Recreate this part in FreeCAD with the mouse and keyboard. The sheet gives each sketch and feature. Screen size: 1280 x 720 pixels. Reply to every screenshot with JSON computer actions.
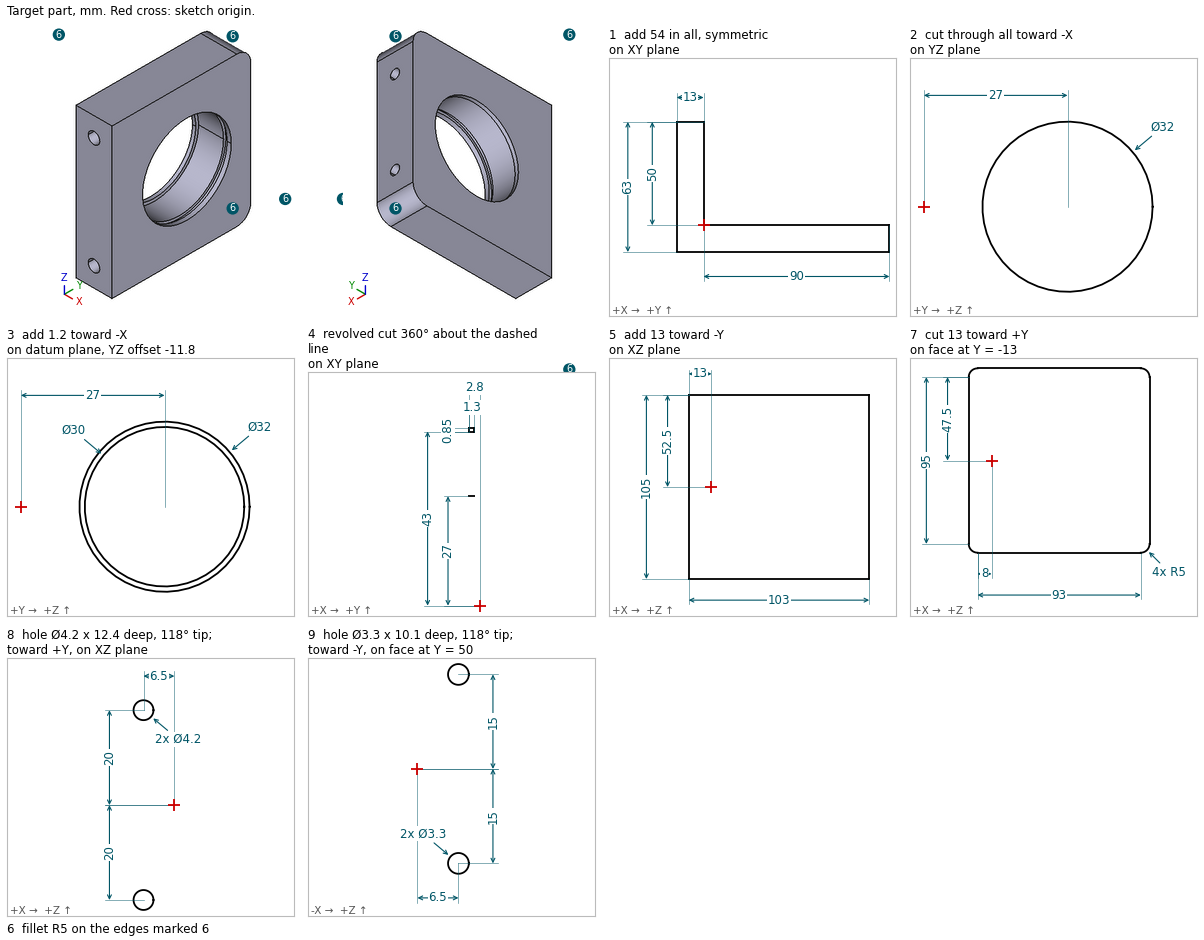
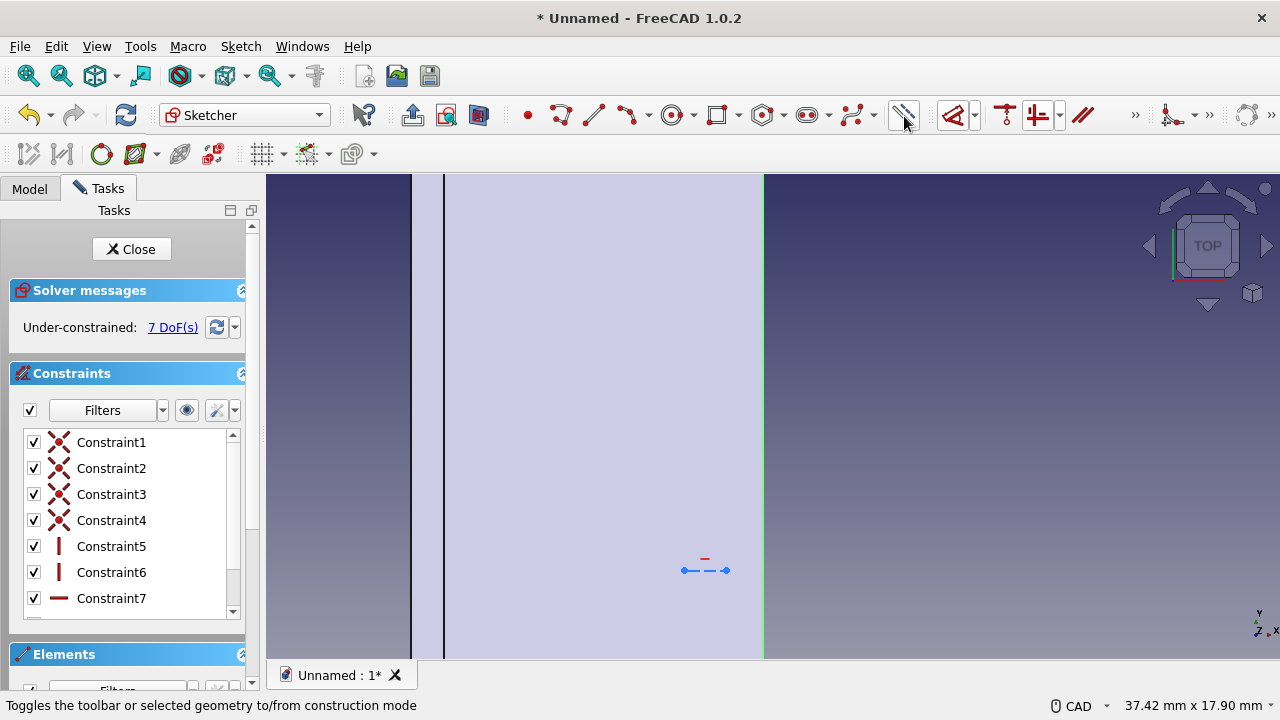
{"action": "scroll", "coordinate": [703, 571], "scroll_direction": "down", "scroll_amount": 2}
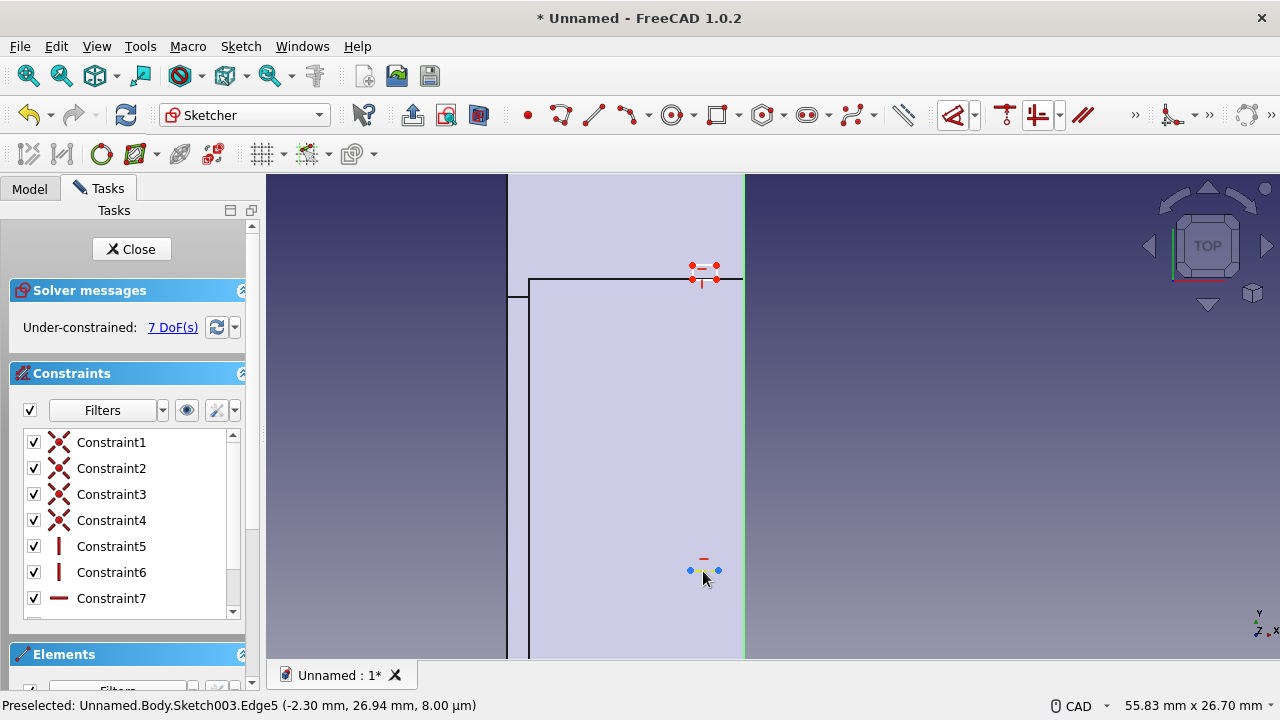
{"action": "scroll", "coordinate": [700, 280], "scroll_direction": "up", "scroll_amount": 4}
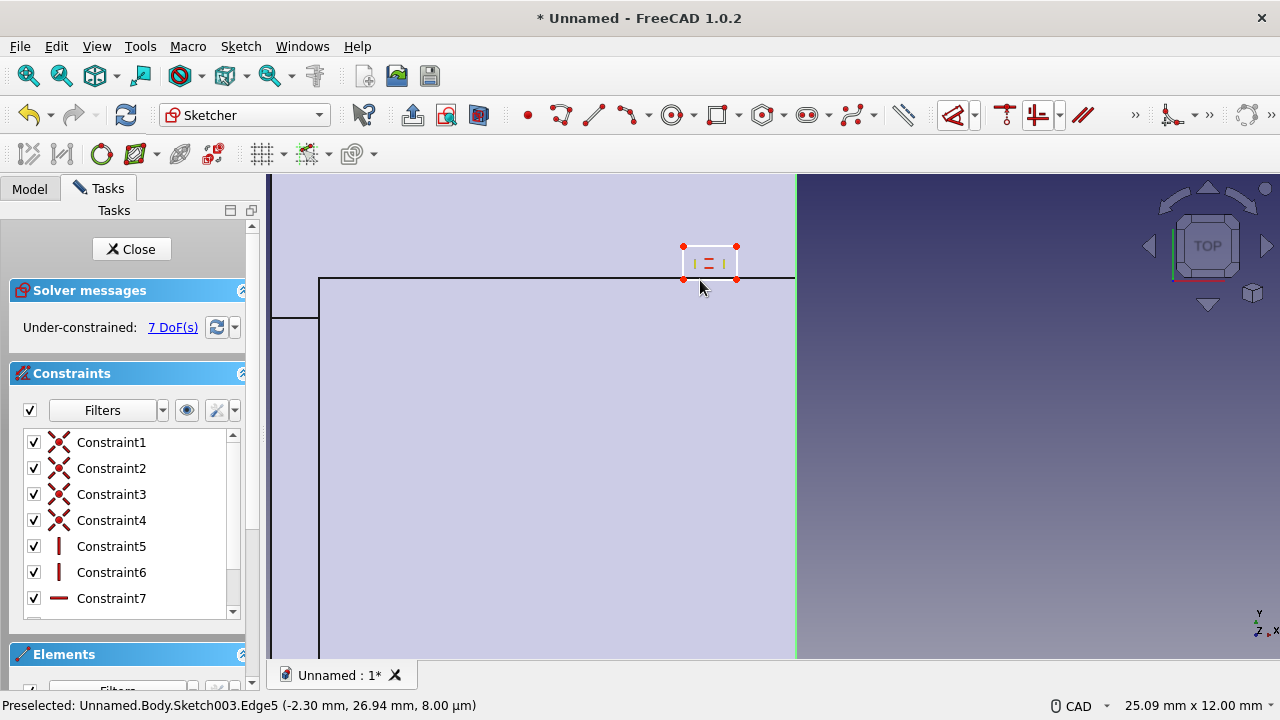
{"action": "left_click", "coordinate": [699, 280]}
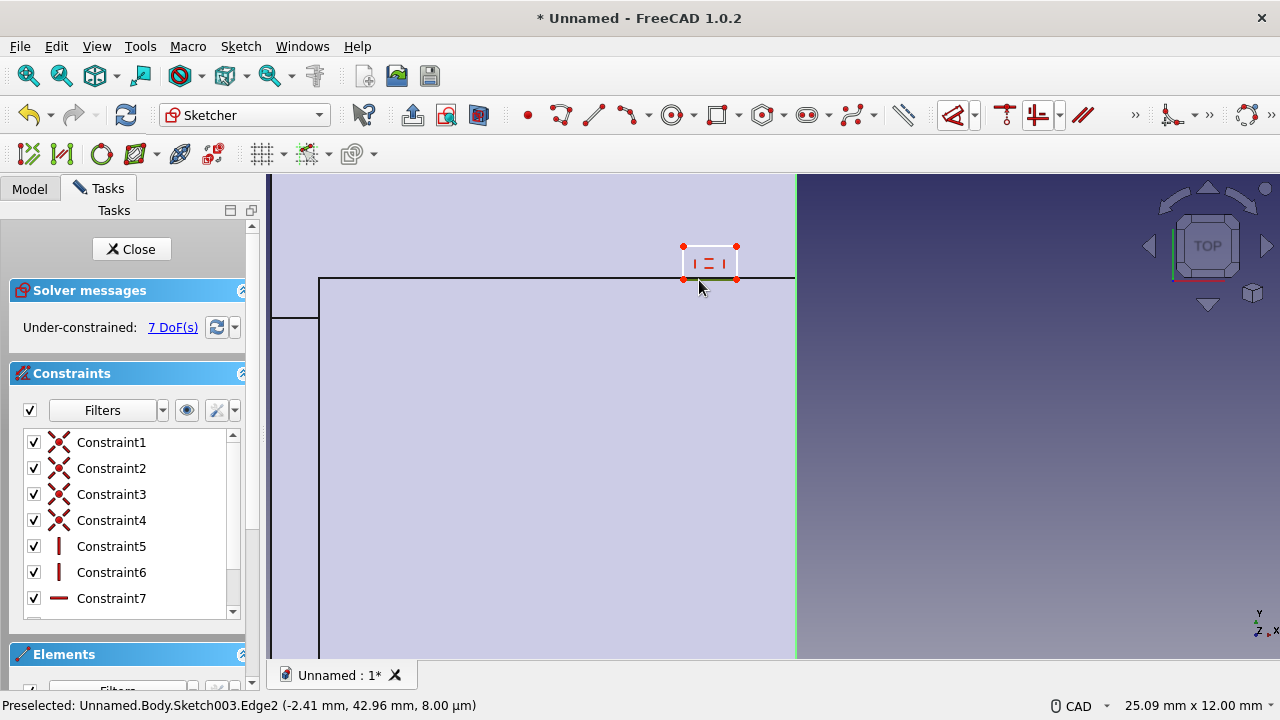
{"action": "left_click", "coordinate": [974, 116]}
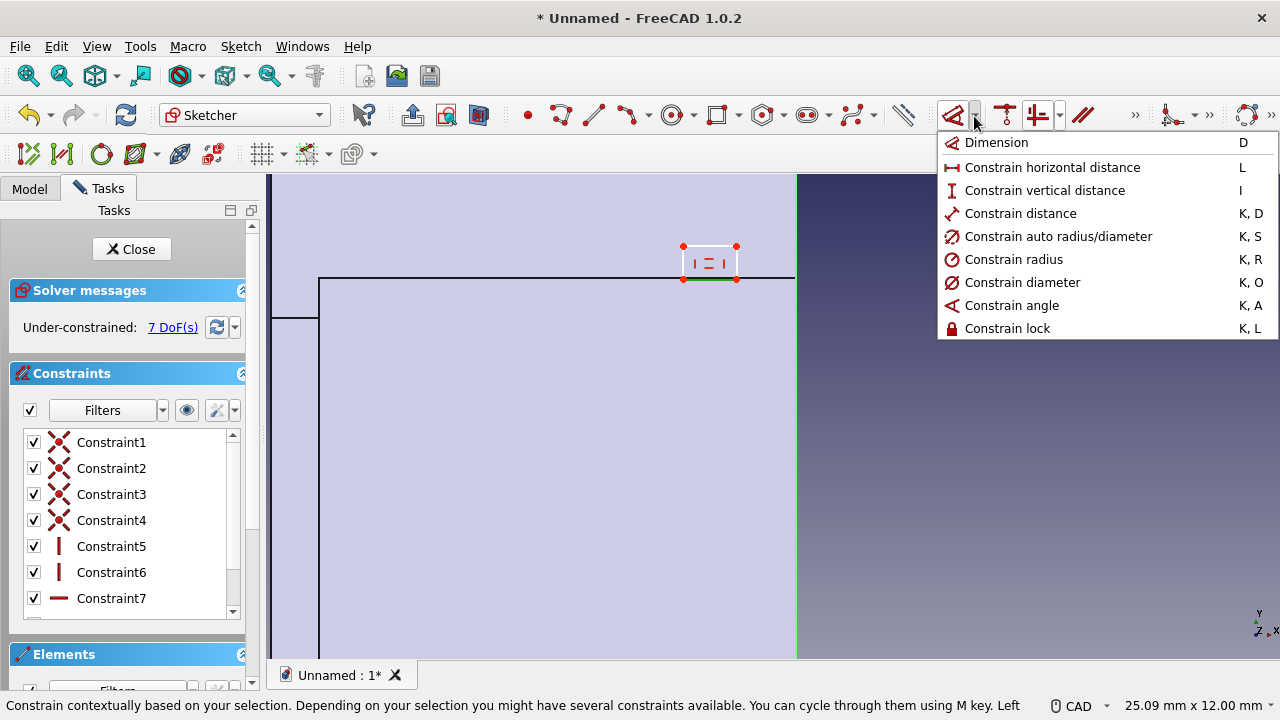
{"action": "left_click", "coordinate": [1108, 168]}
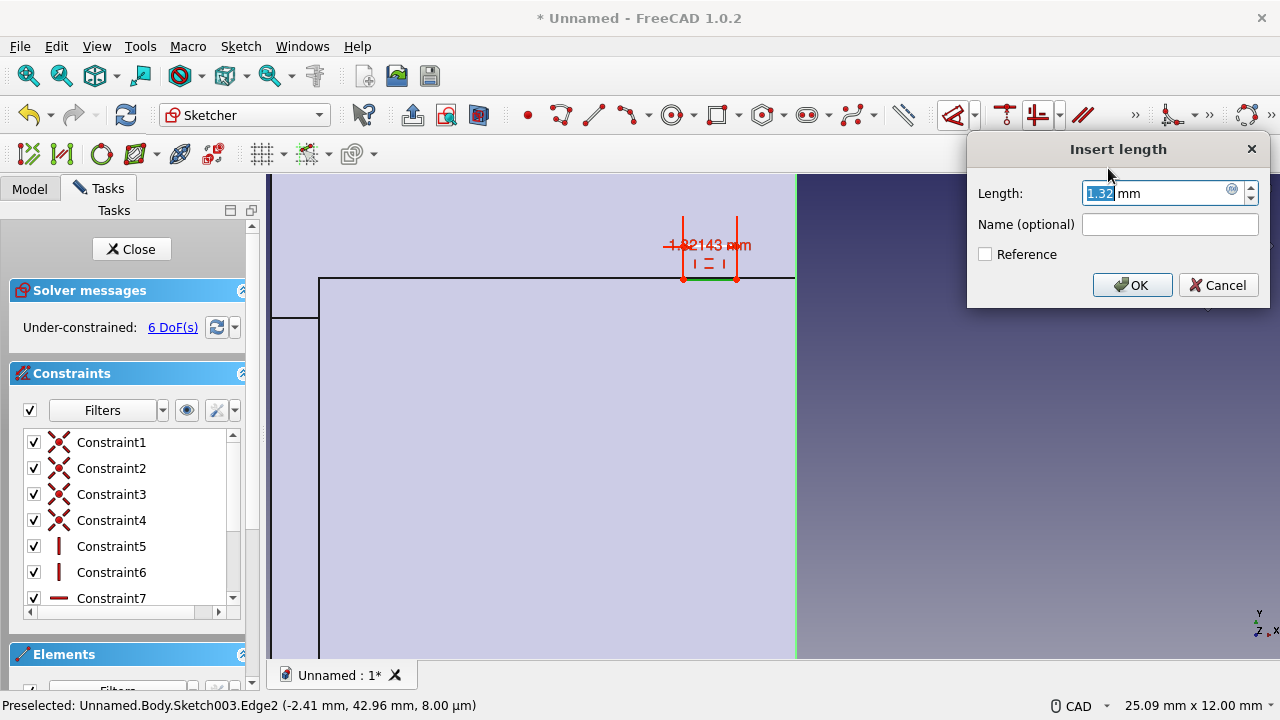
{"action": "type", "text": "1.3"}
{"action": "key", "text": "Return"}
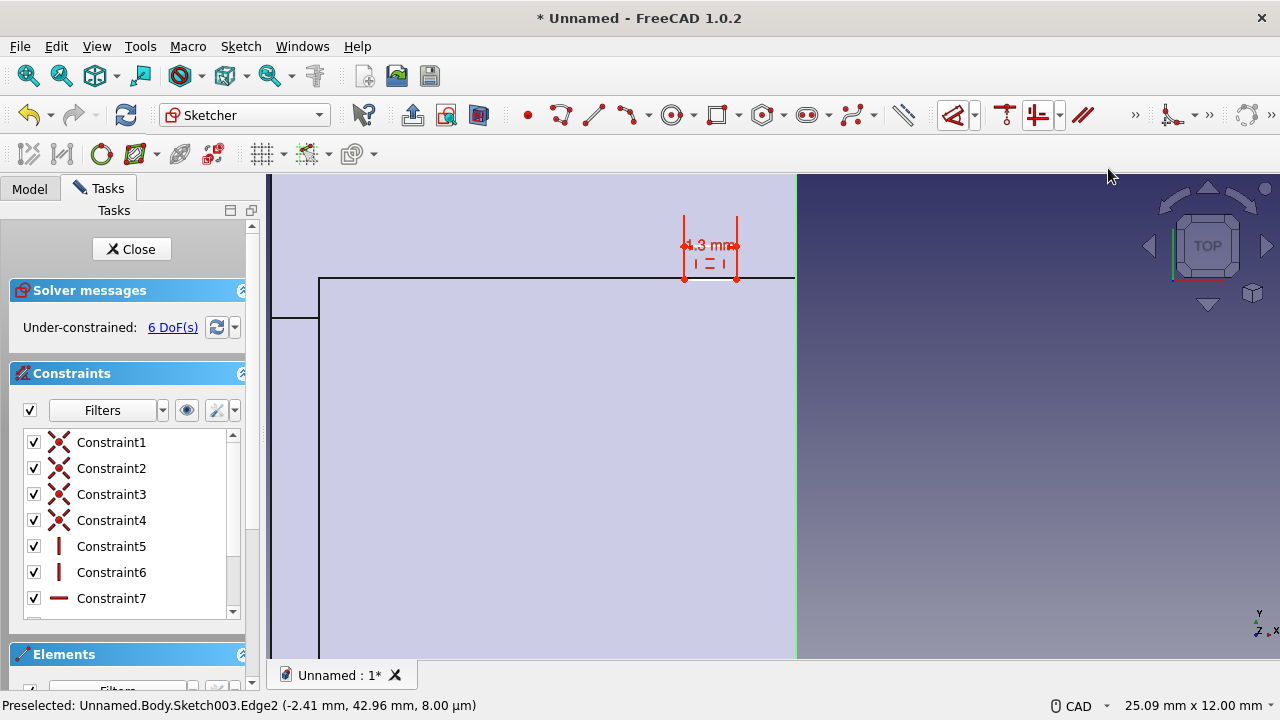
{"action": "left_click", "coordinate": [684, 280]}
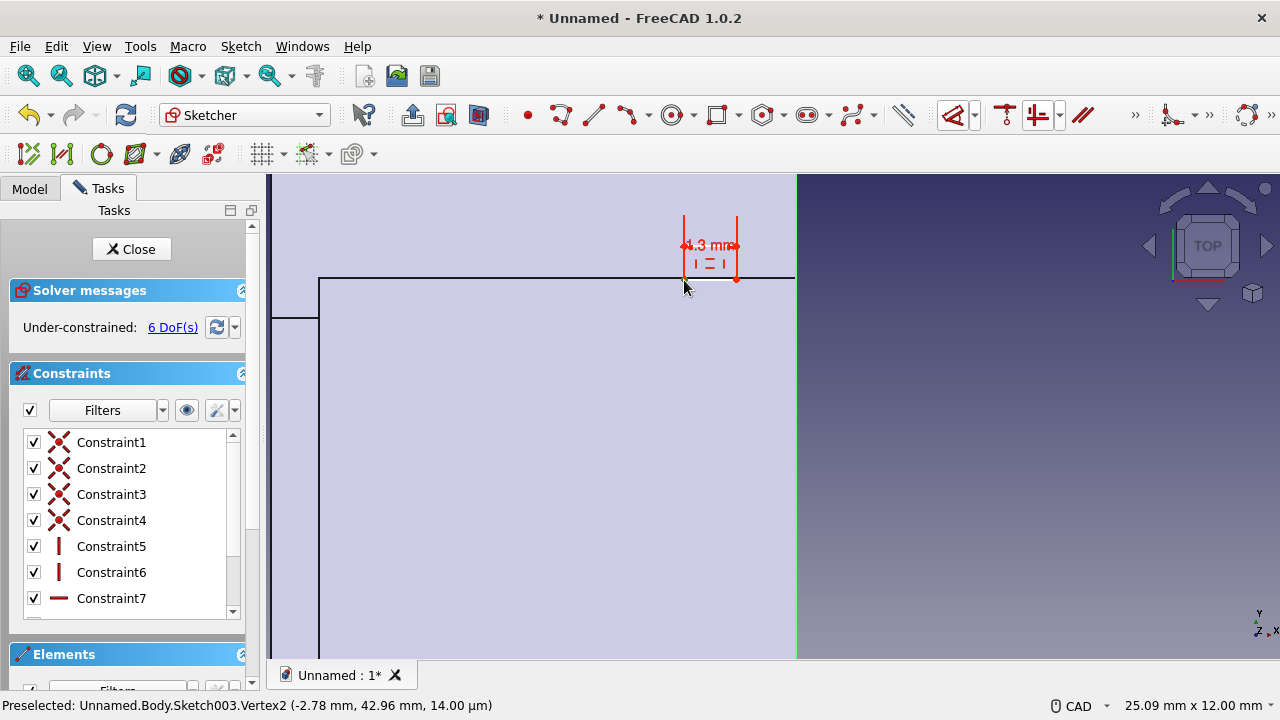
{"action": "left_click", "coordinate": [974, 116]}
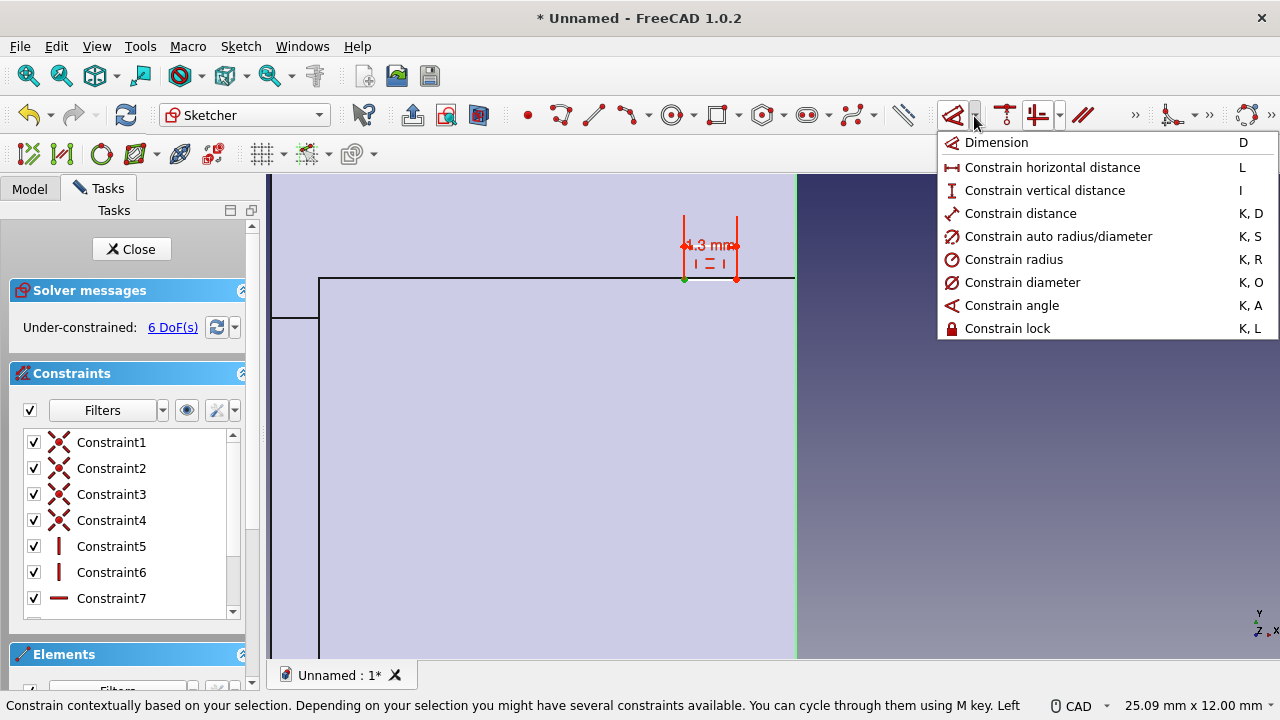
{"action": "left_click", "coordinate": [1108, 190]}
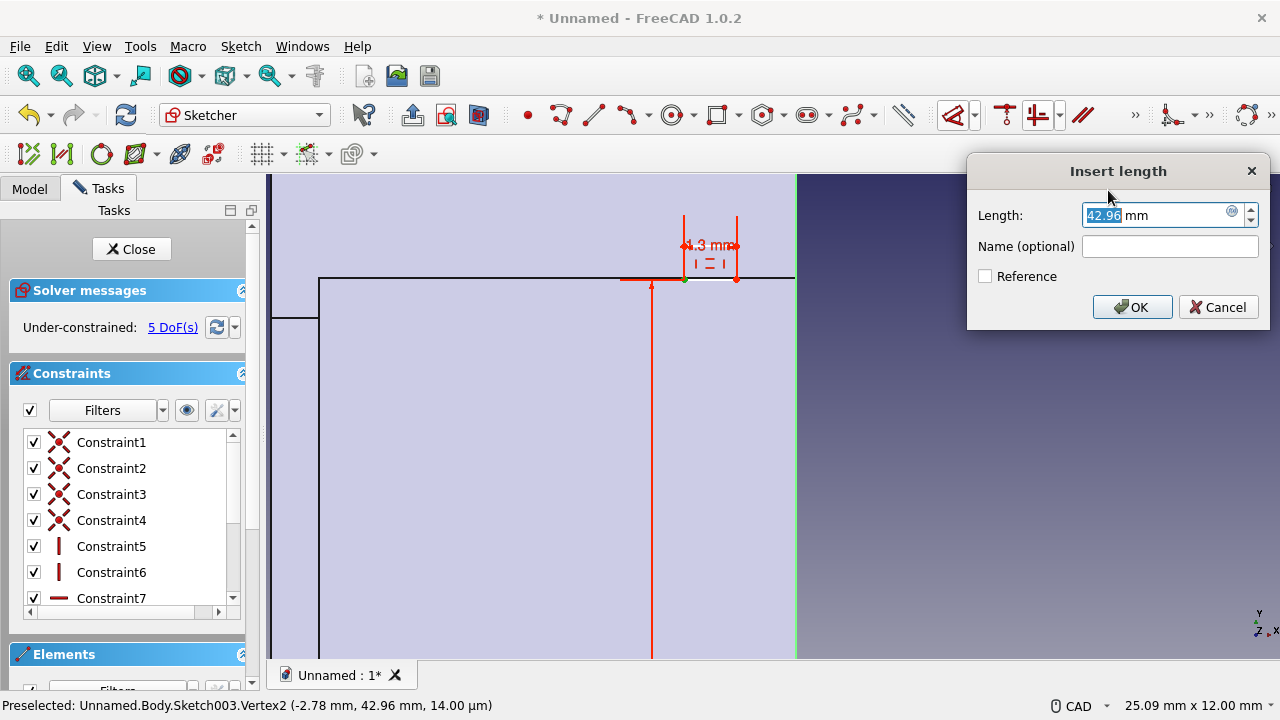
{"action": "type", "text": "43"}
{"action": "key", "text": "Return"}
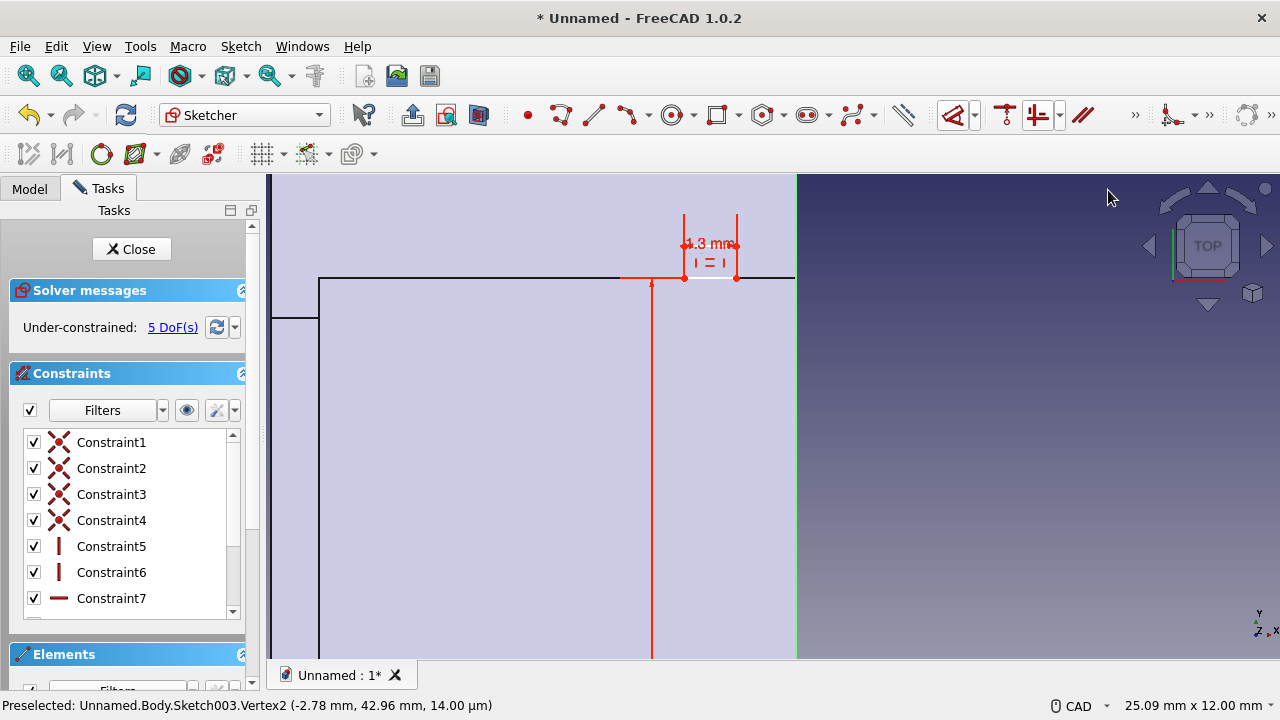
{"action": "scroll", "coordinate": [700, 280], "scroll_direction": "down", "scroll_amount": 4}